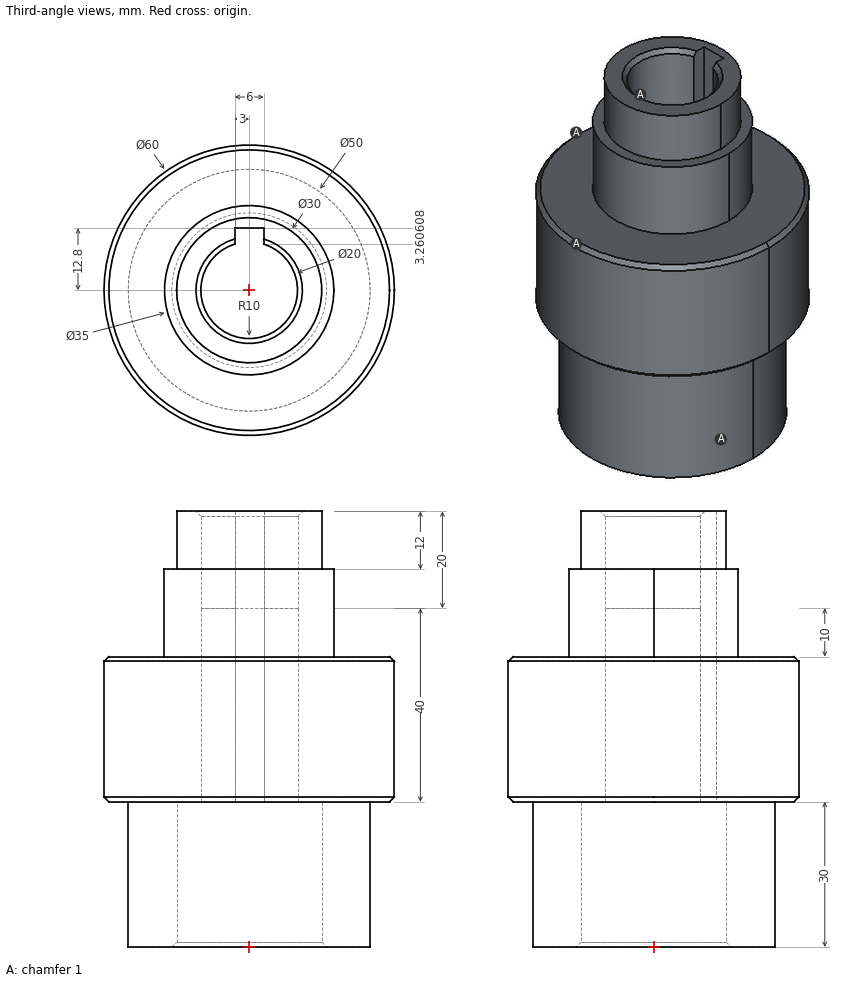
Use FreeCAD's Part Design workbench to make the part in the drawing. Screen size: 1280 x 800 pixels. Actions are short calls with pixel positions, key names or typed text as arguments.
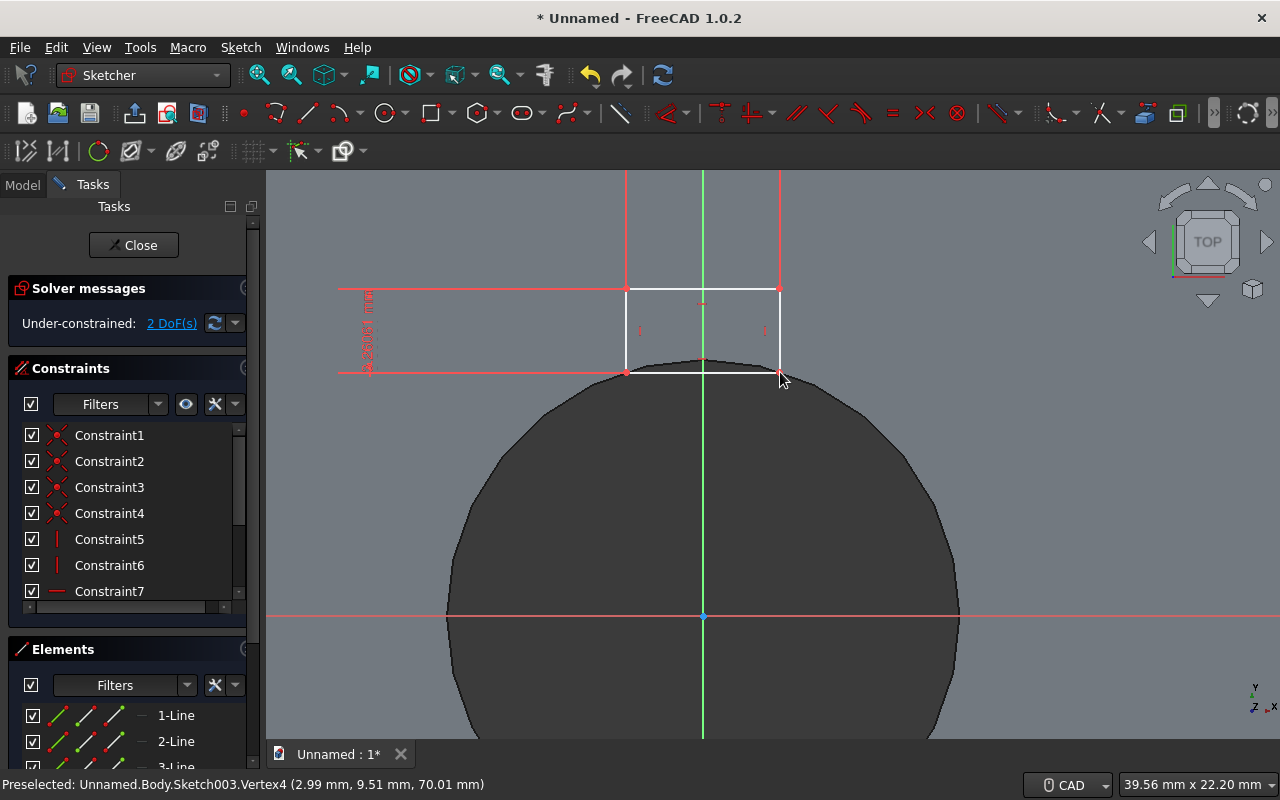
click(666, 114)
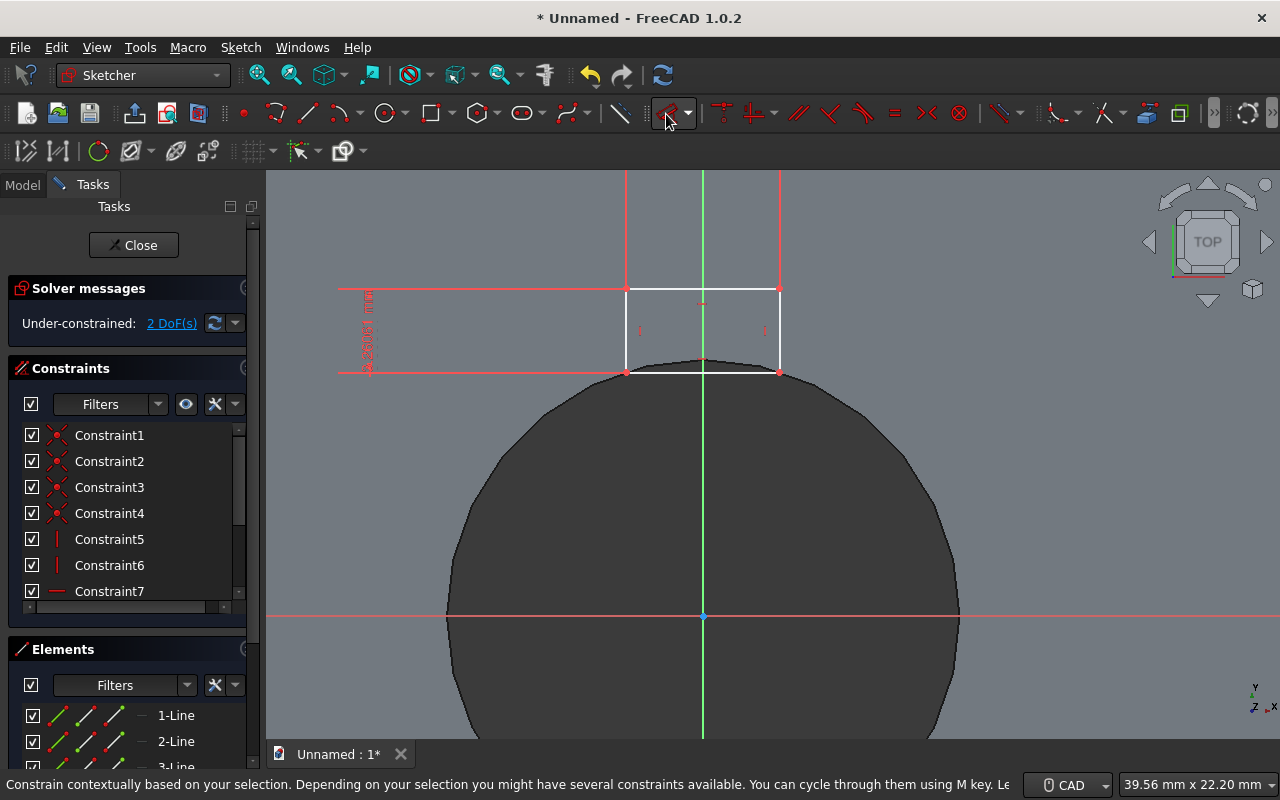
click(626, 289)
click(665, 650)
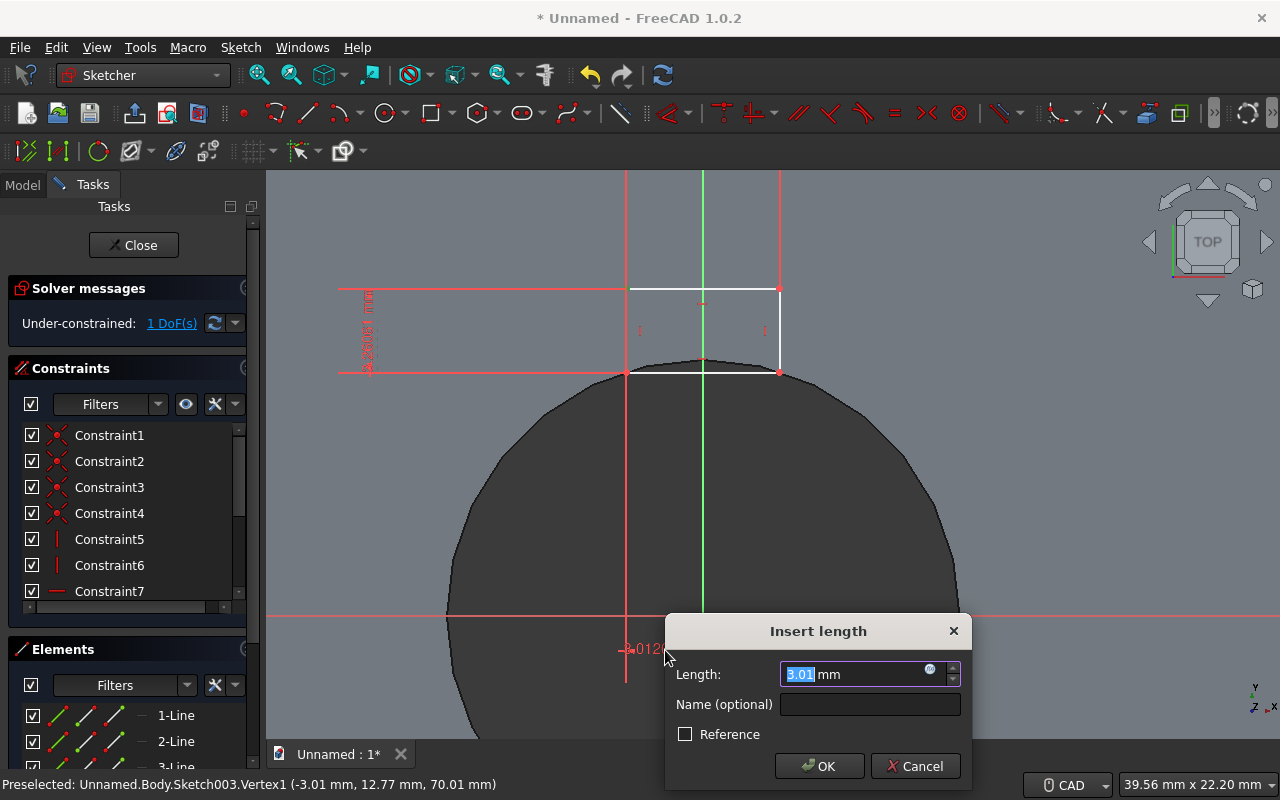
text(3)
key(Return)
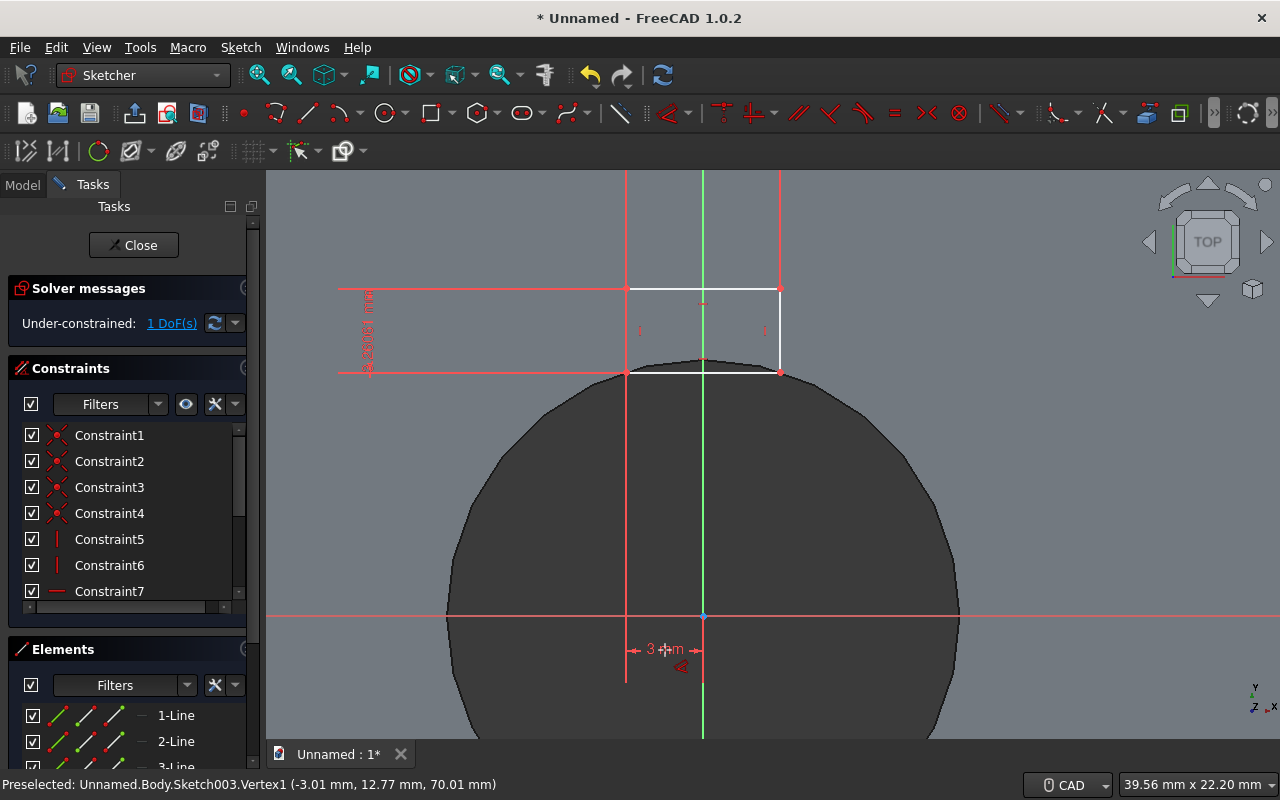
click(626, 289)
click(592, 453)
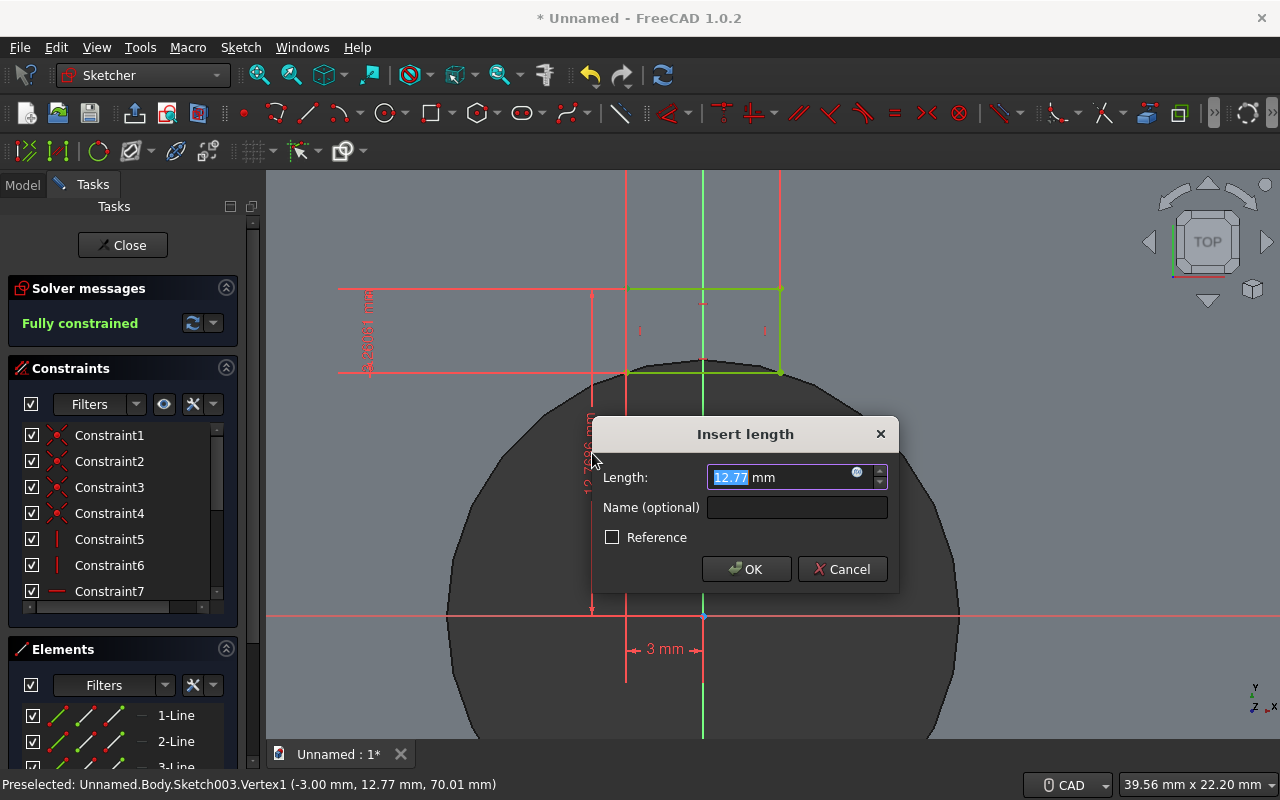
text(12.8)
key(Return)
key(Escape)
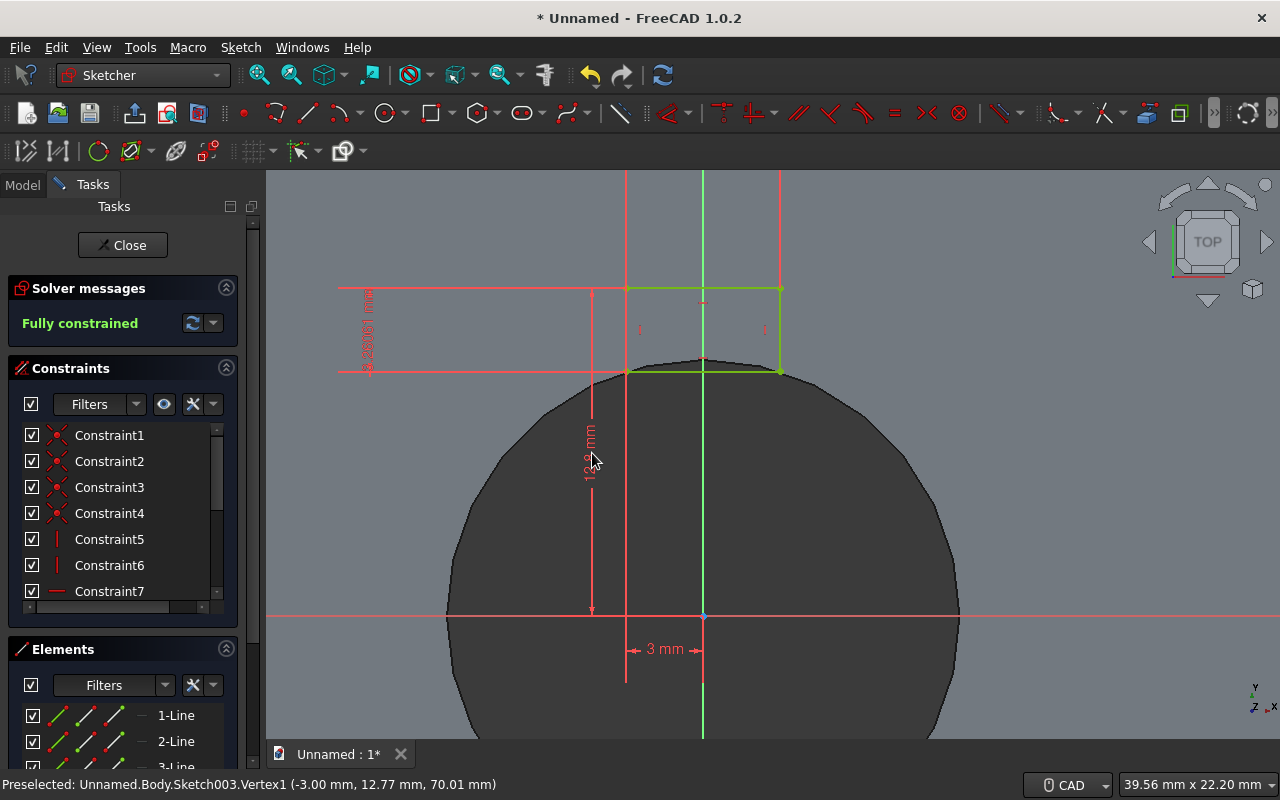
click(123, 245)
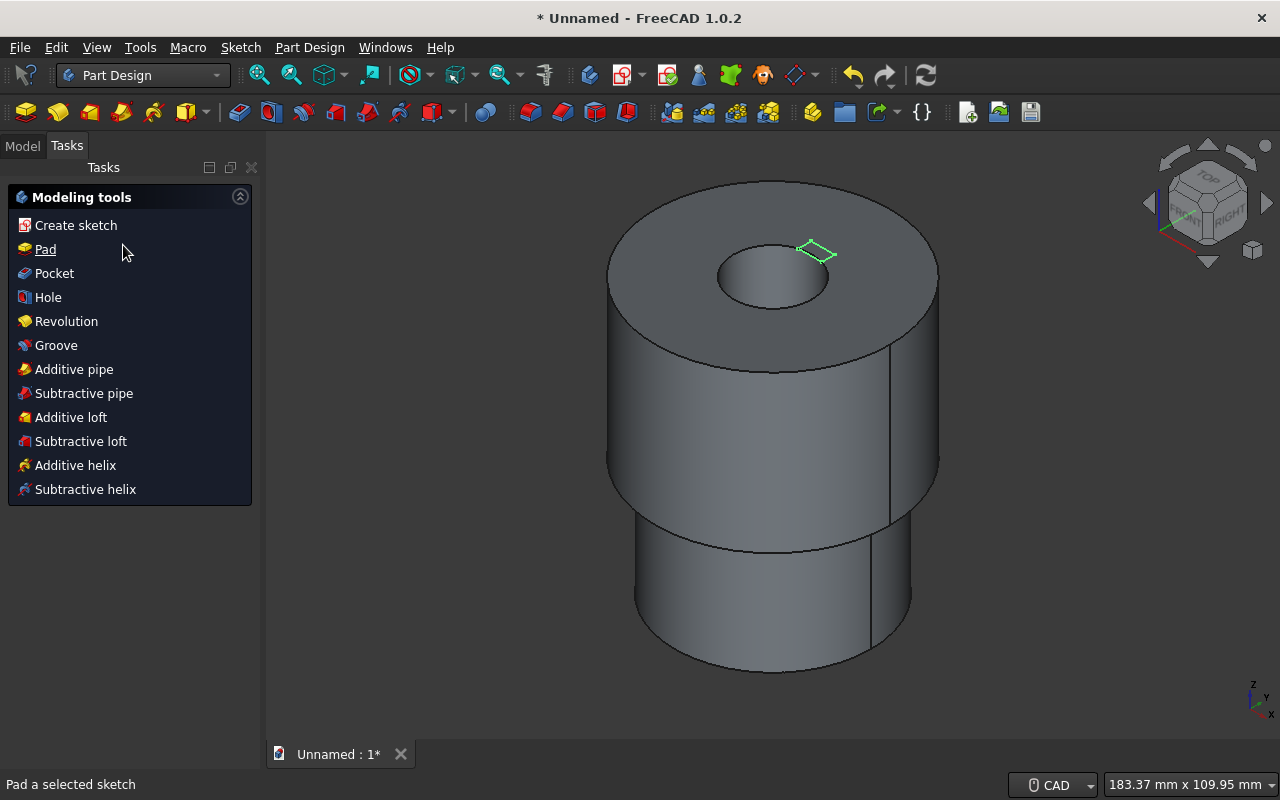
click(240, 112)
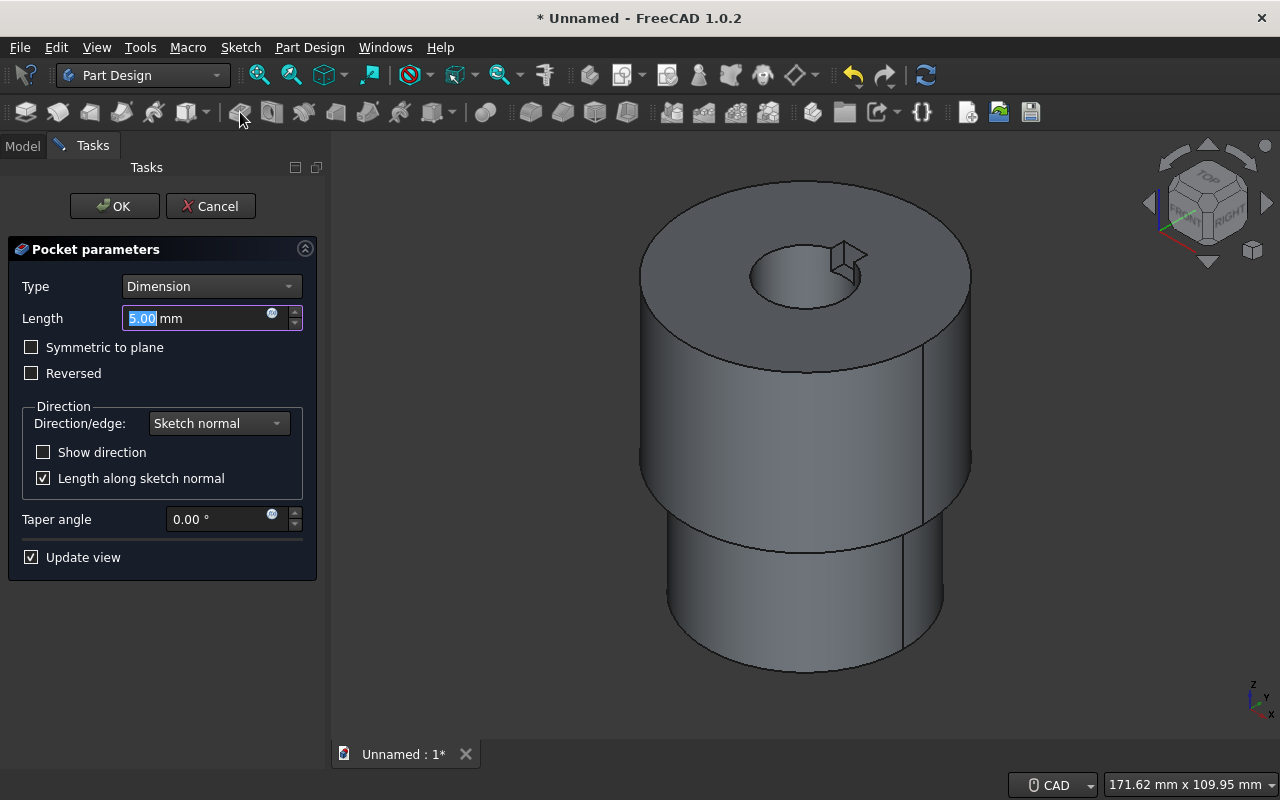
click(212, 286)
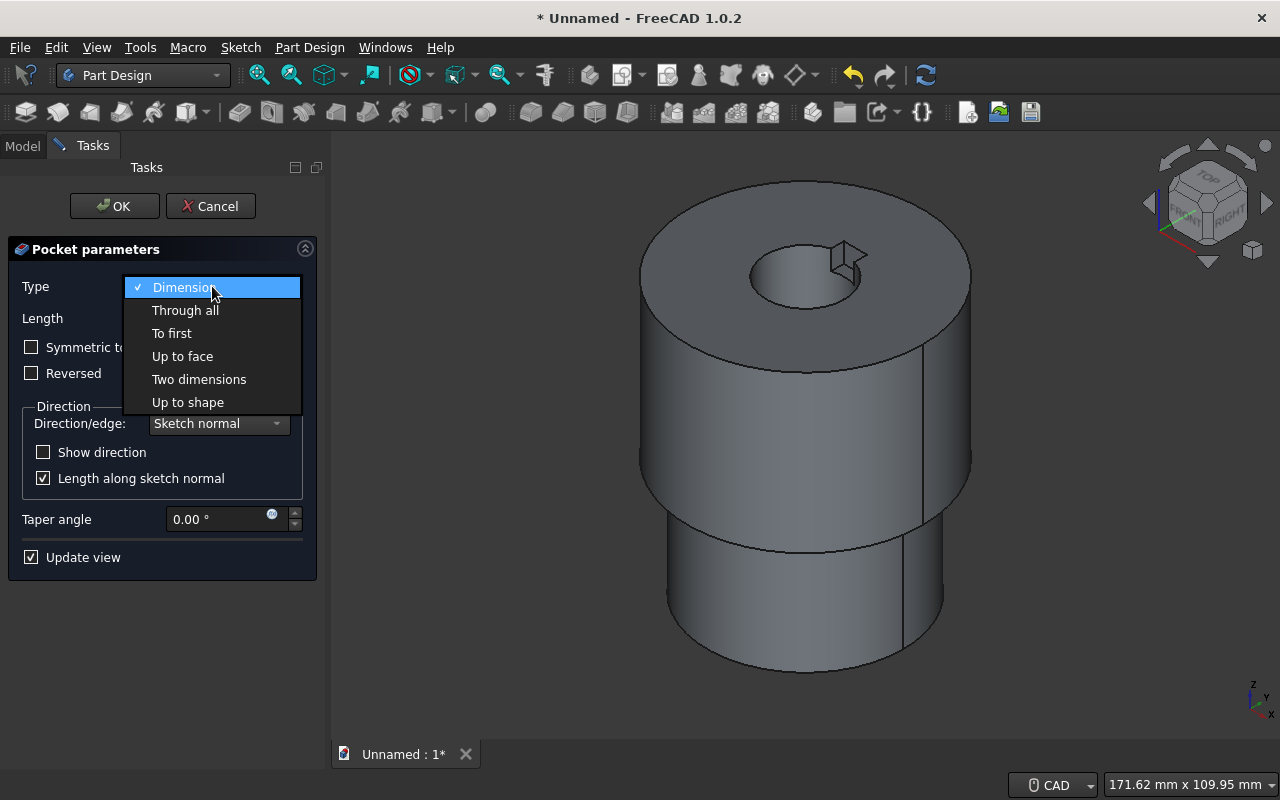
click(212, 310)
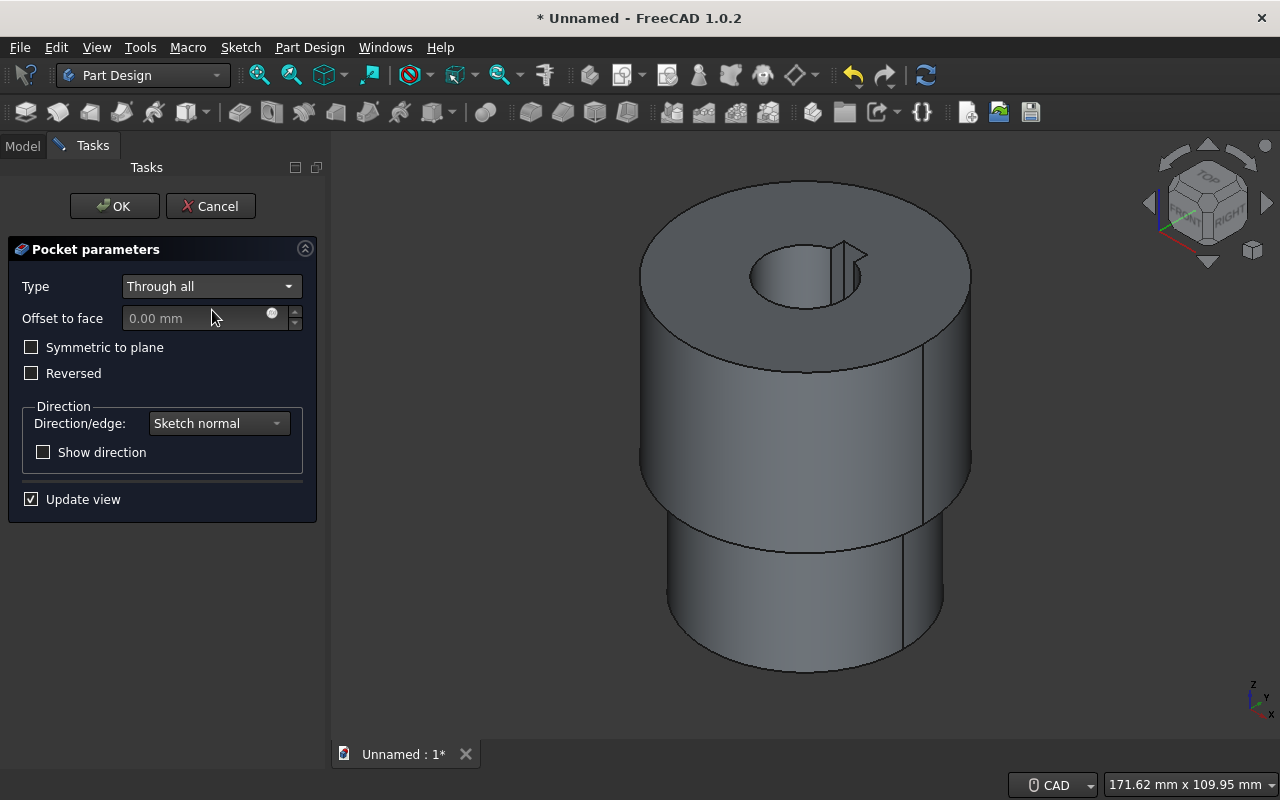
click(115, 206)